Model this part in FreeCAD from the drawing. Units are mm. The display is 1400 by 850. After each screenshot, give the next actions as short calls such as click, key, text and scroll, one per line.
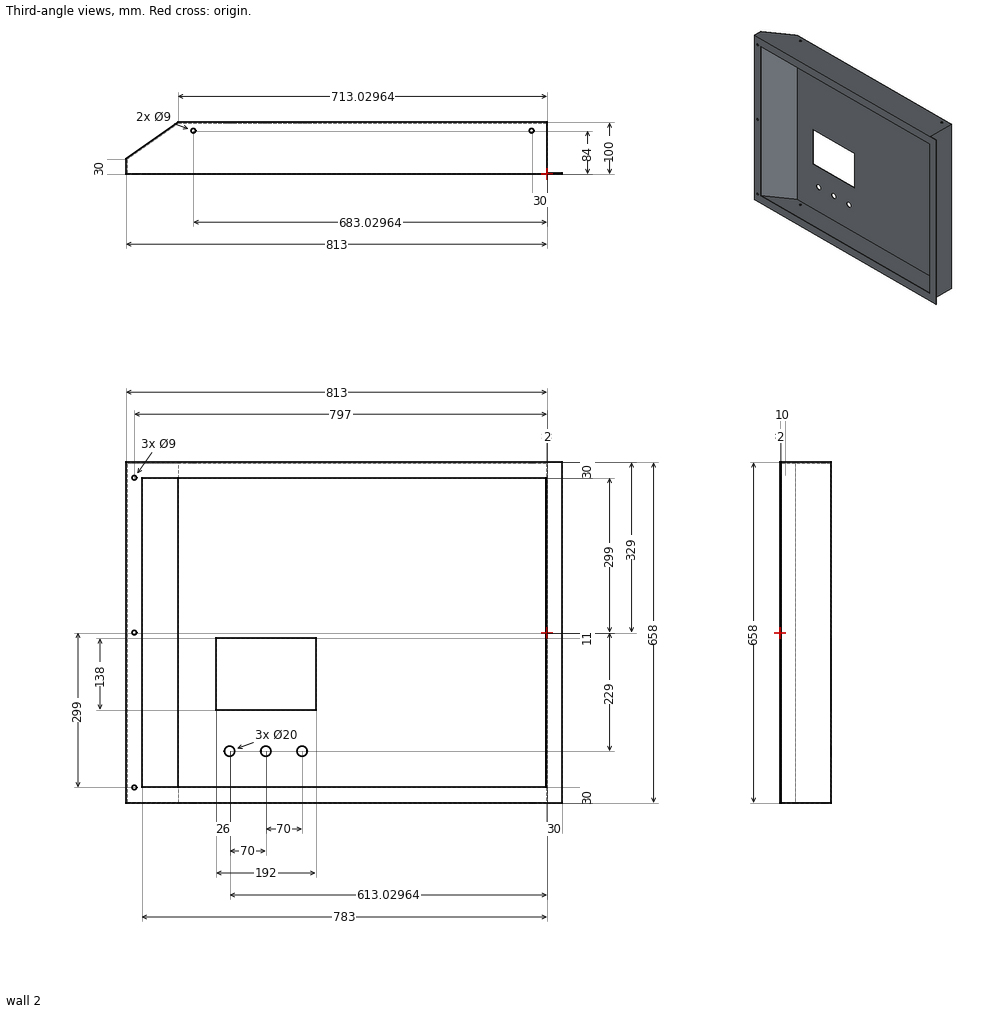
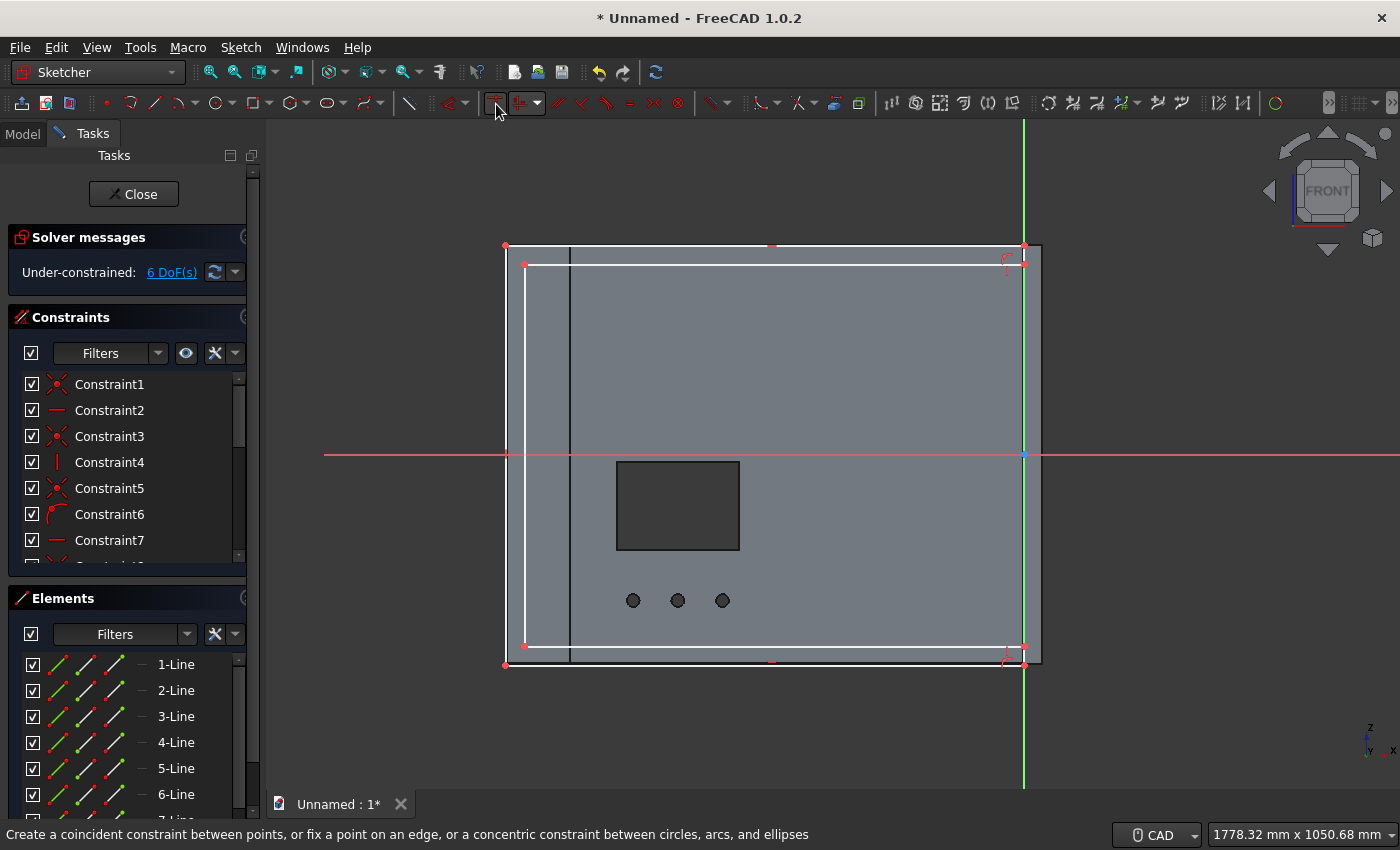
click(448, 104)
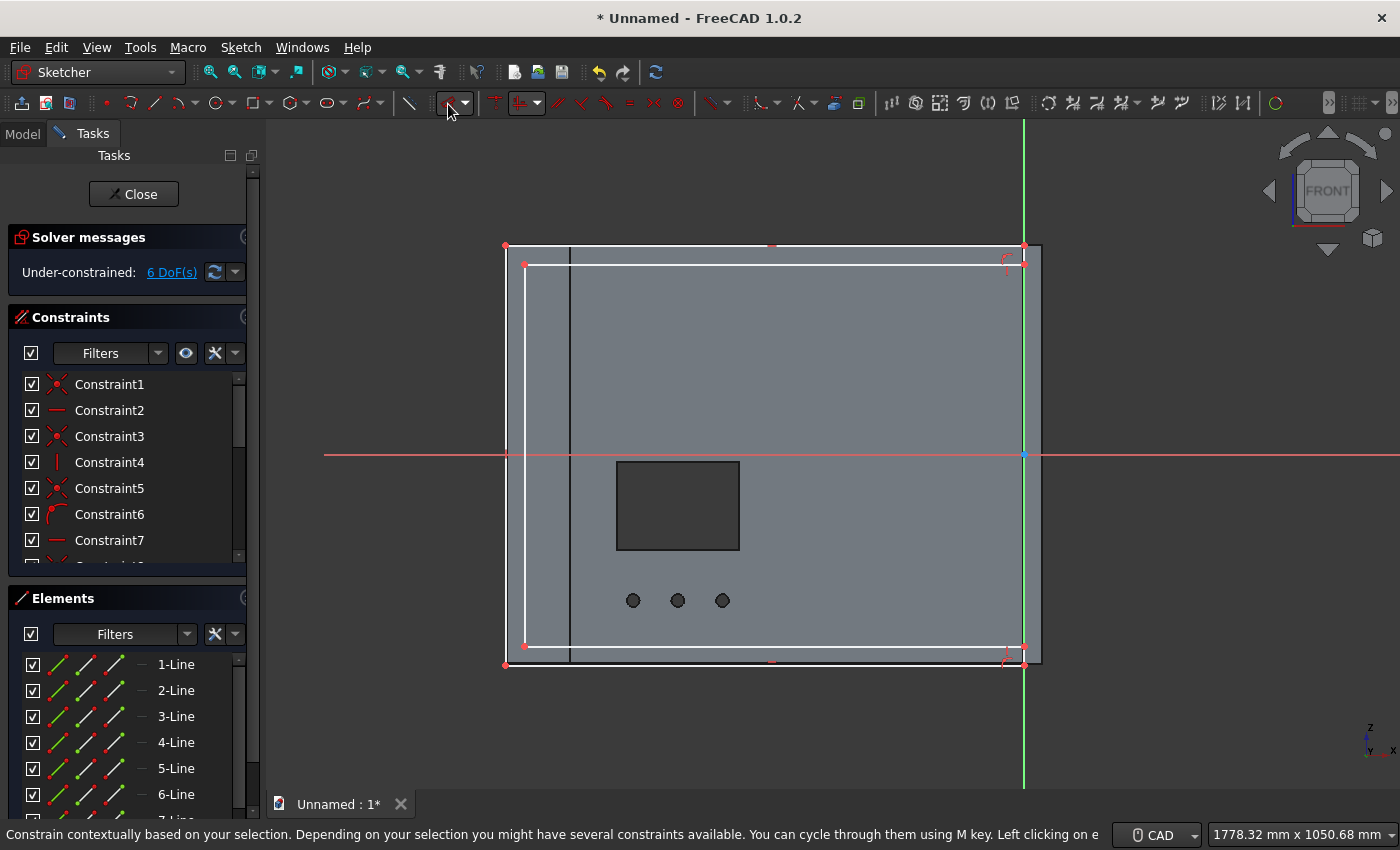
scroll(1024, 255, up, 4)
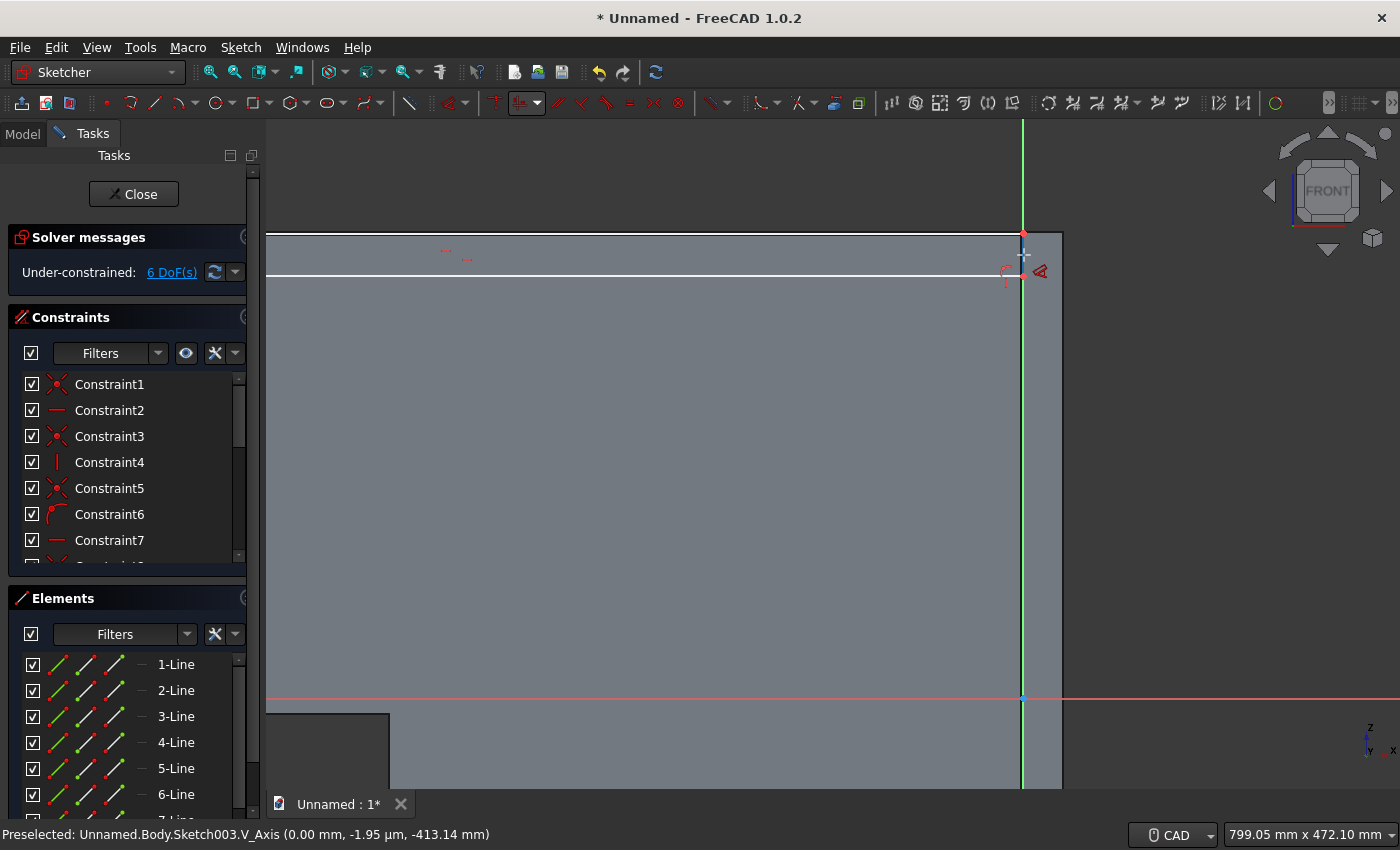
click(1023, 255)
click(1057, 255)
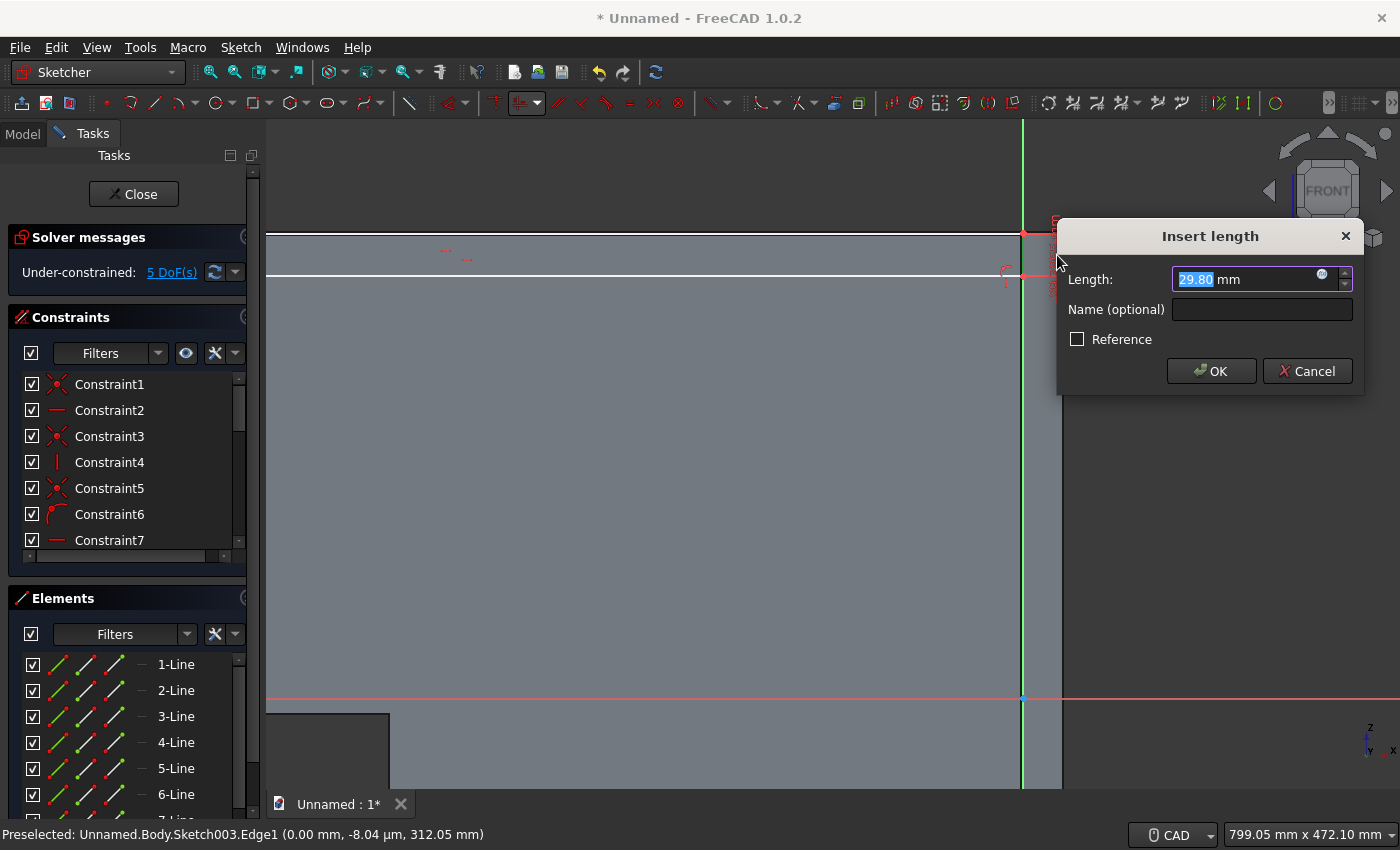
text(30)
key(Return)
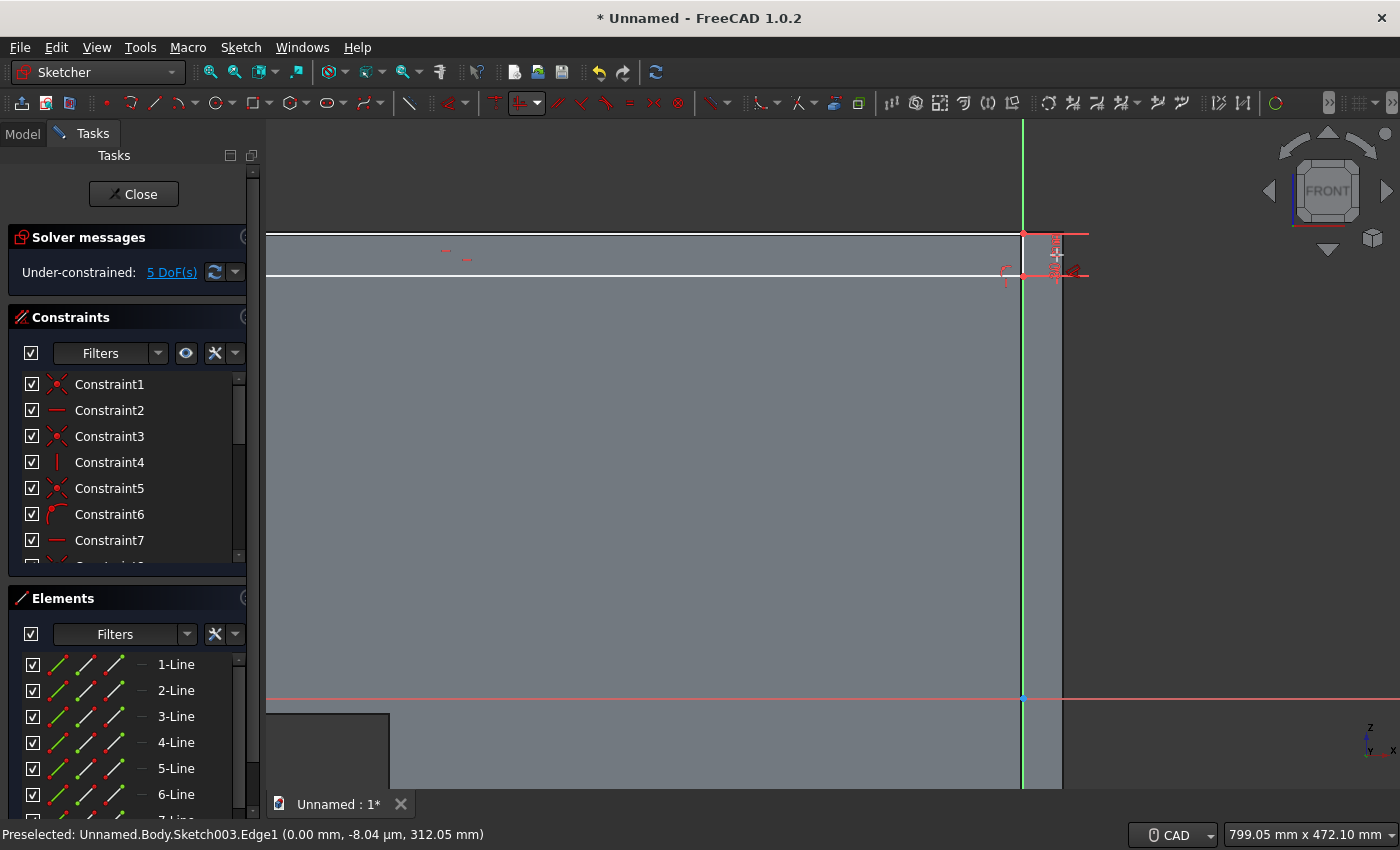
scroll(1024, 254, down, 4)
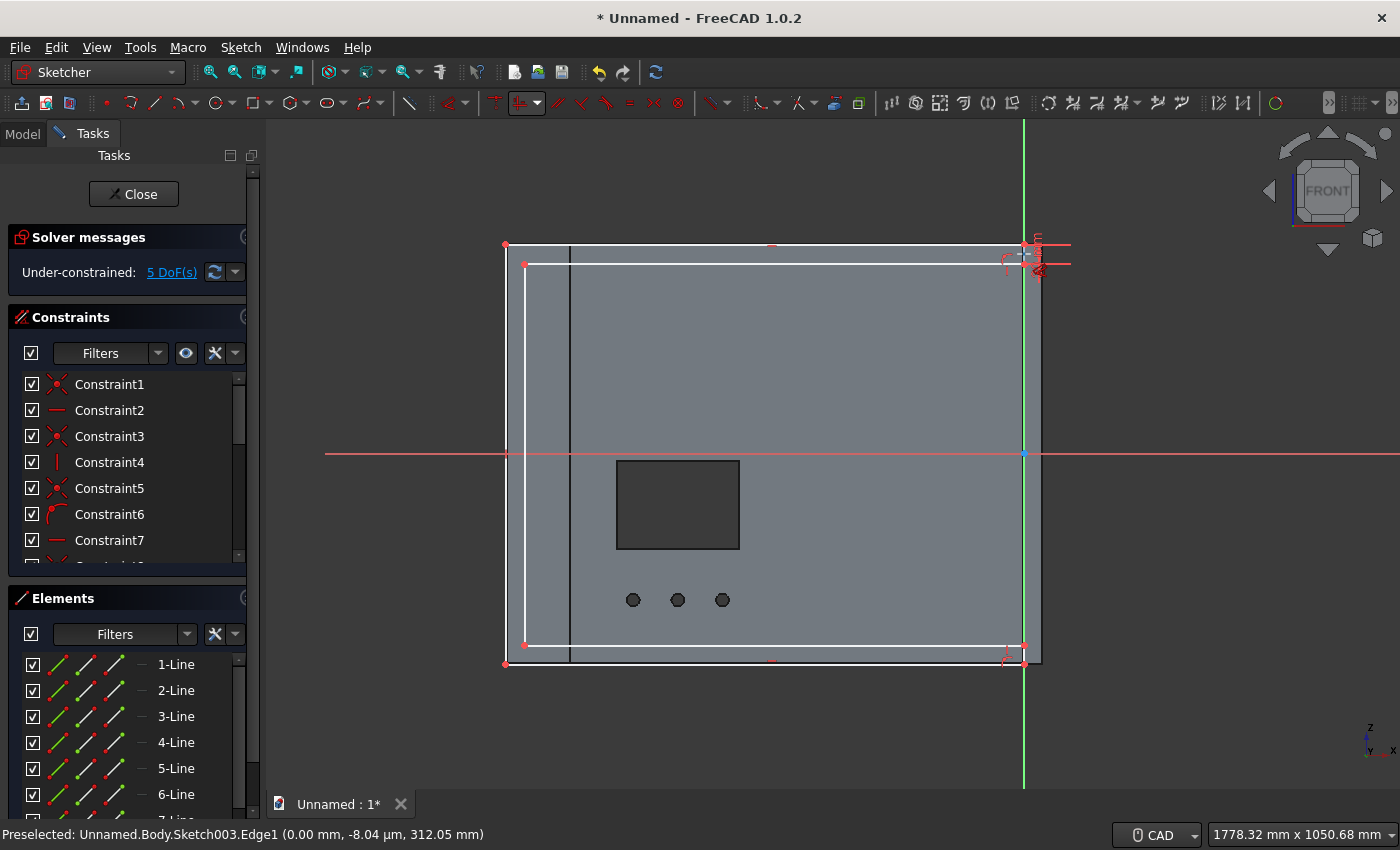
scroll(1024, 659, up, 5)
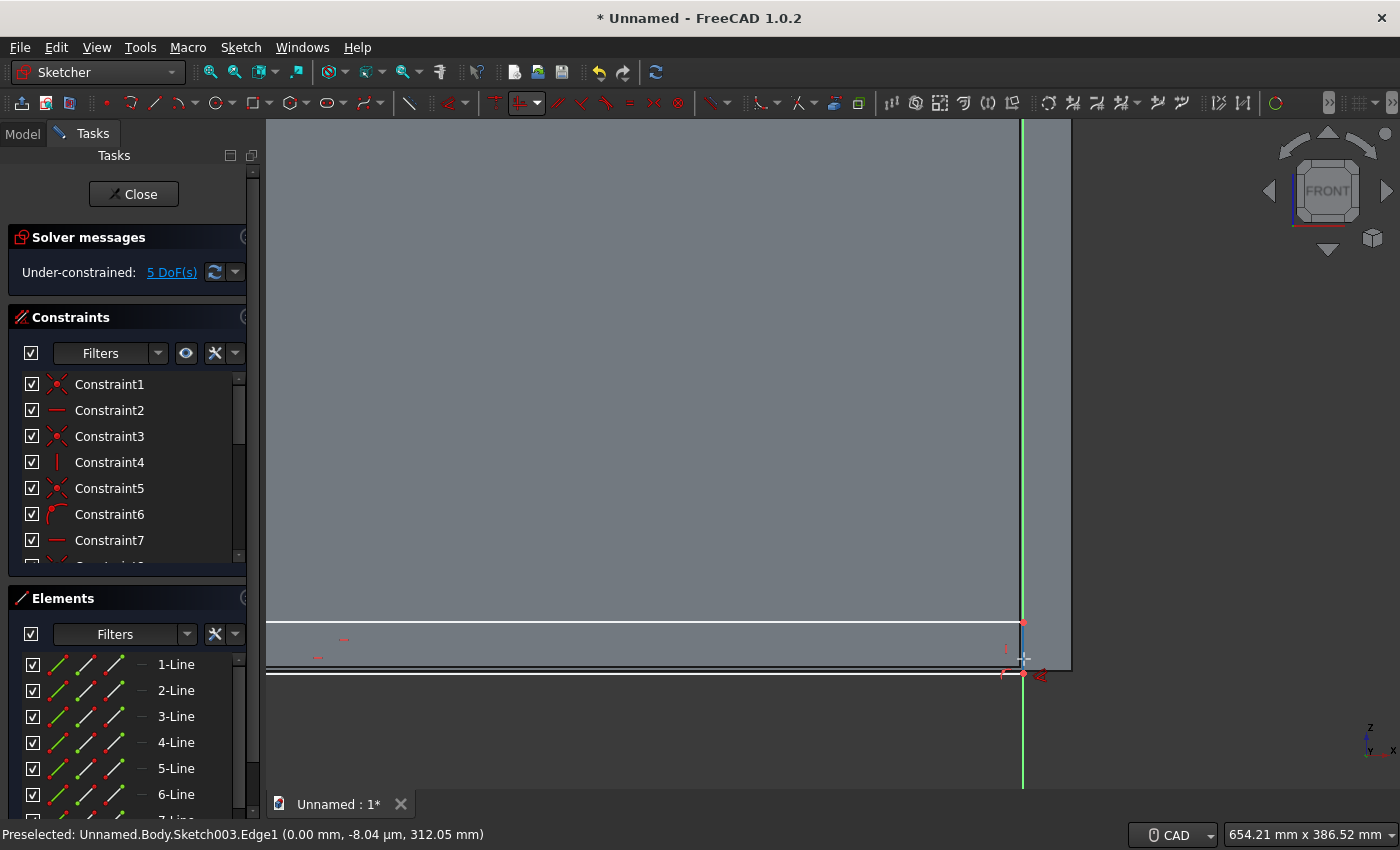
click(1023, 658)
click(1057, 648)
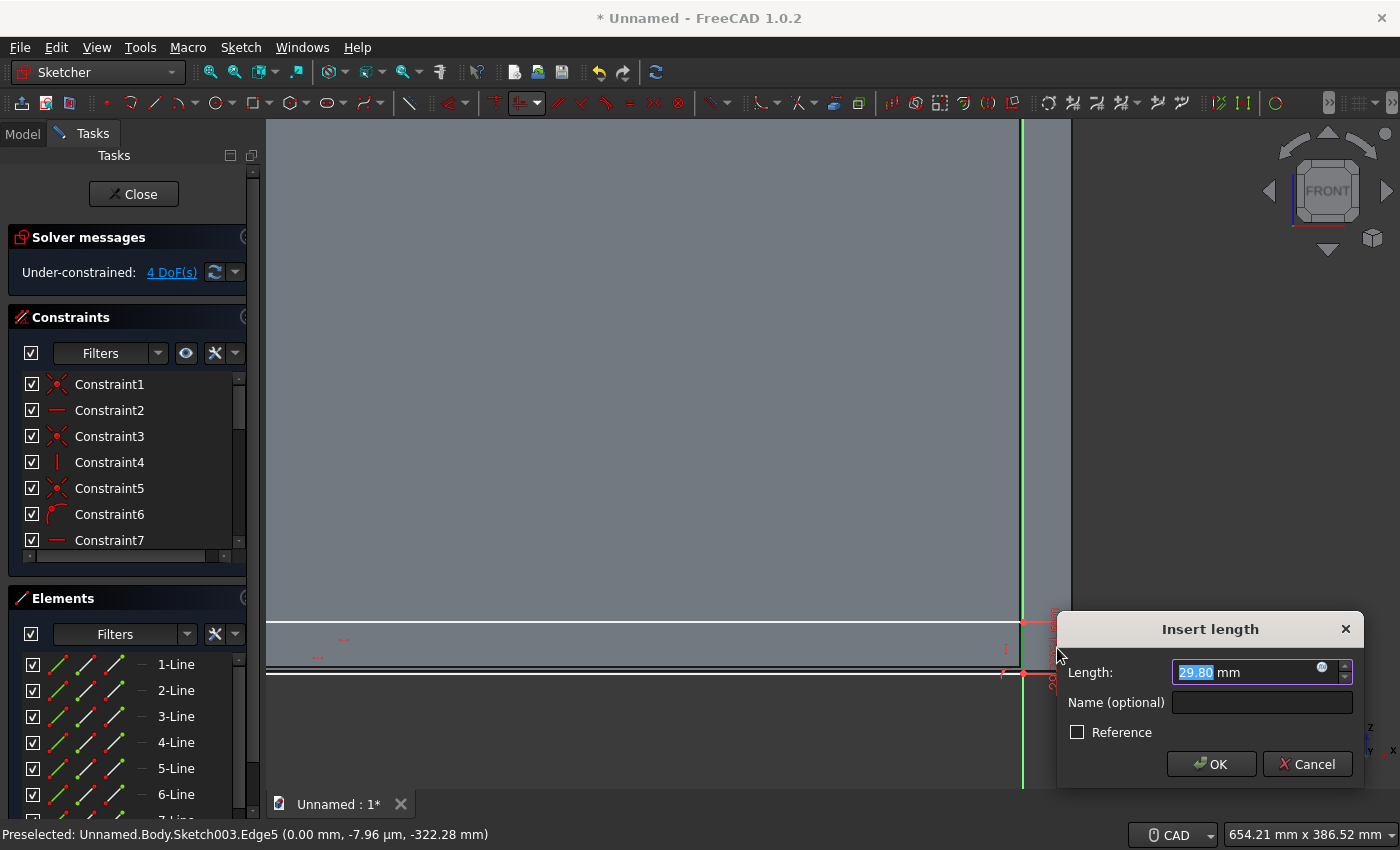
text(30)
key(Return)